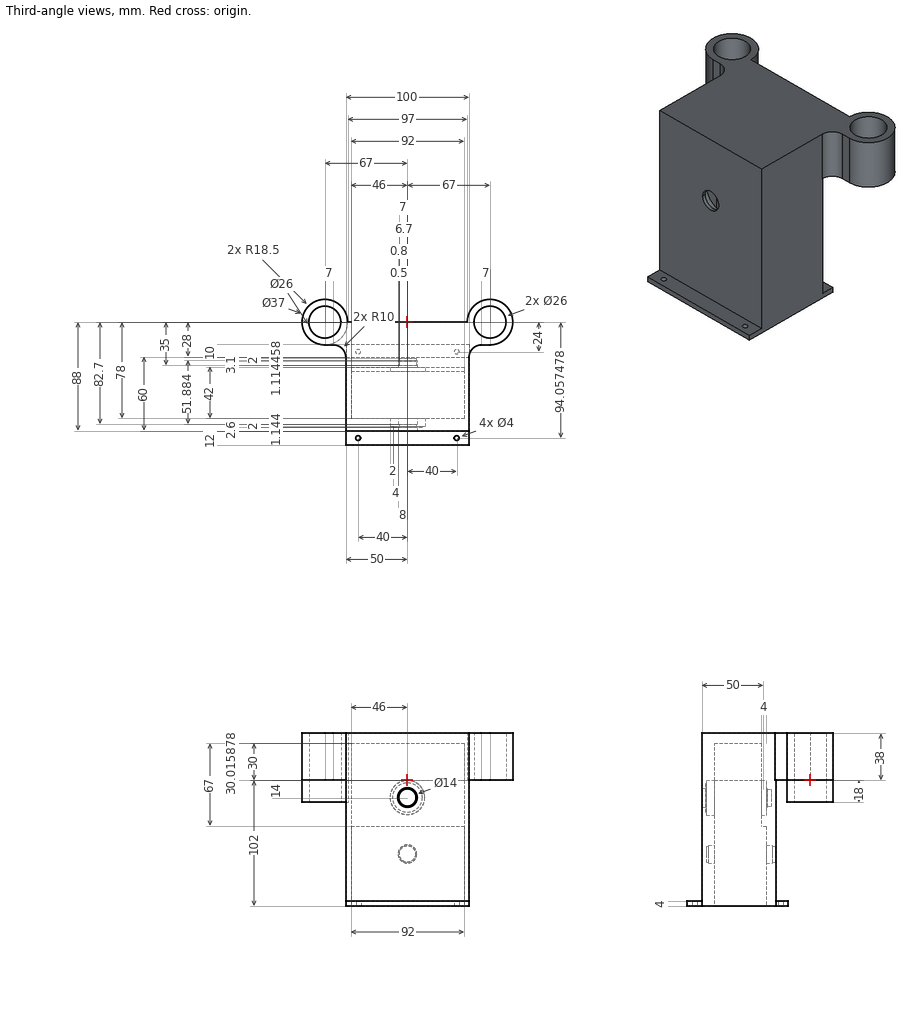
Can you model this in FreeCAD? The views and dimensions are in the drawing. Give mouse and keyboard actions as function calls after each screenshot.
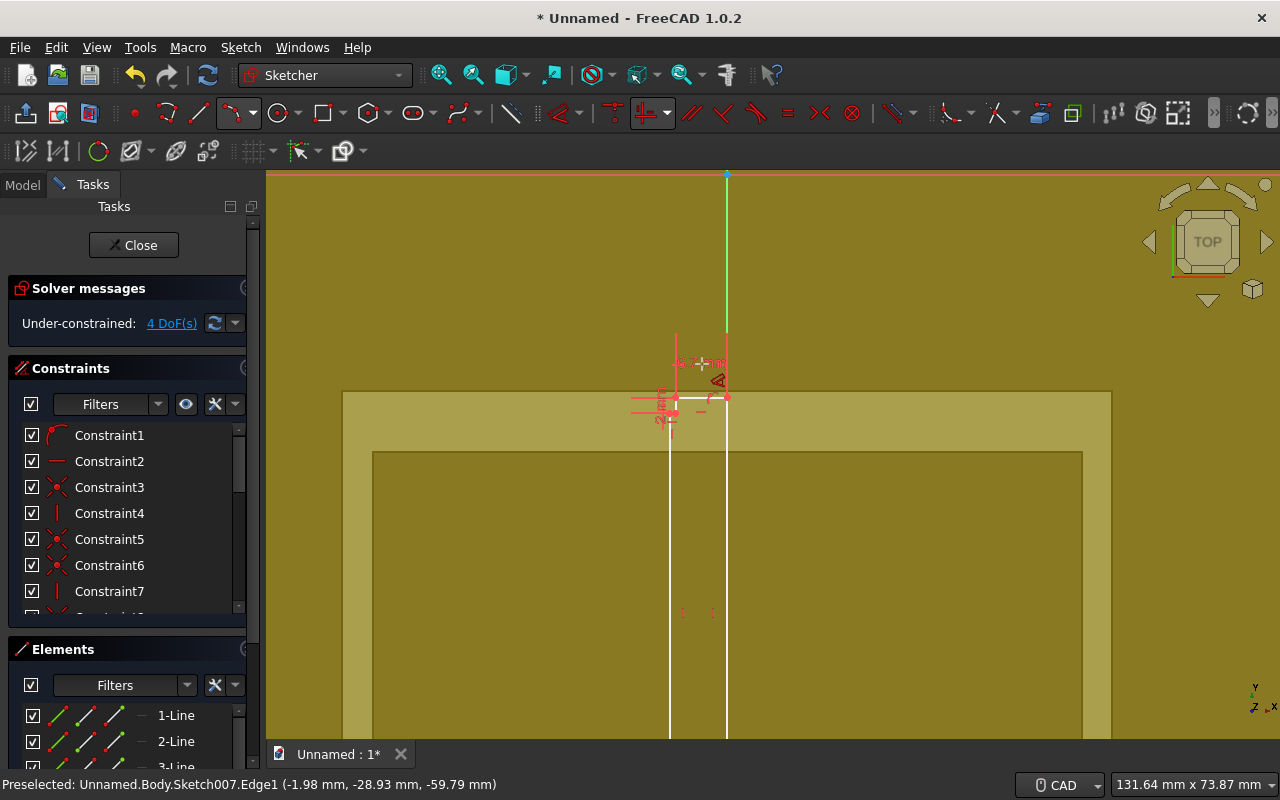
scroll(673, 413, up, 10)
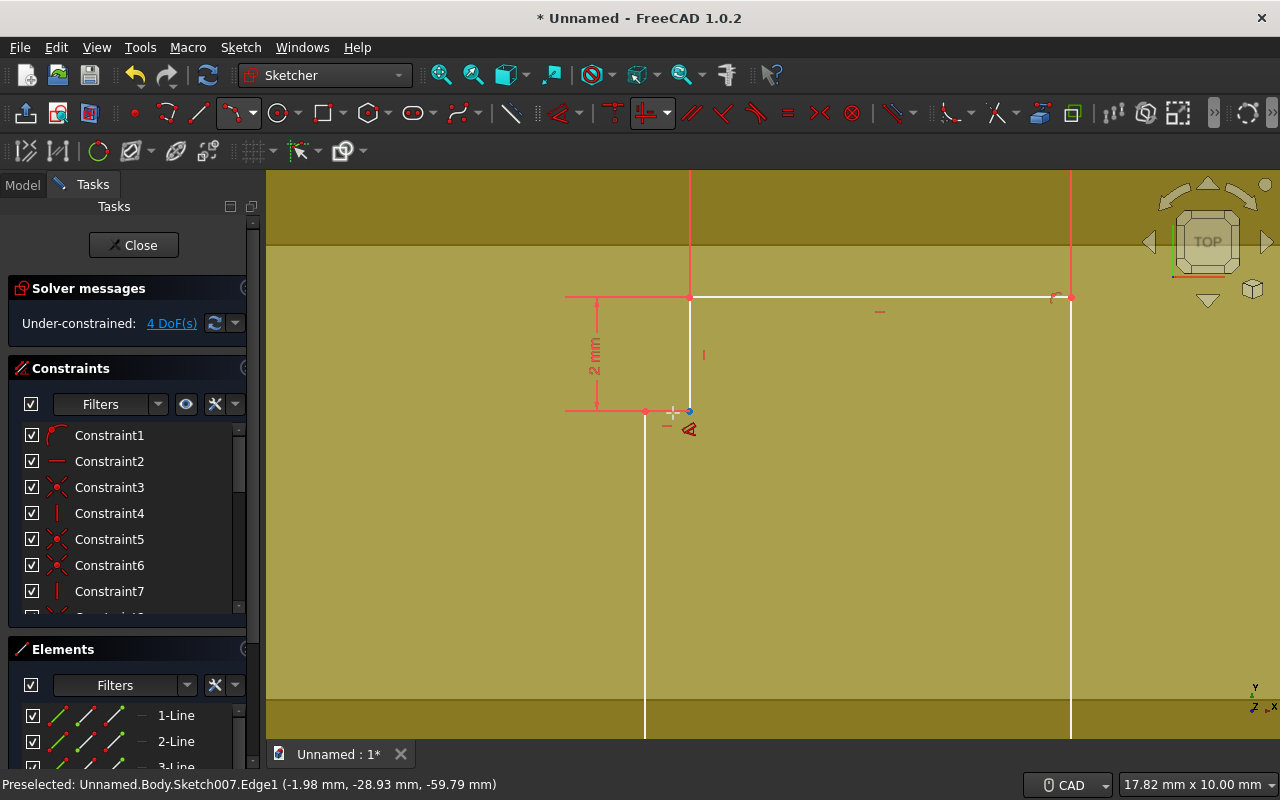
click(668, 411)
click(668, 377)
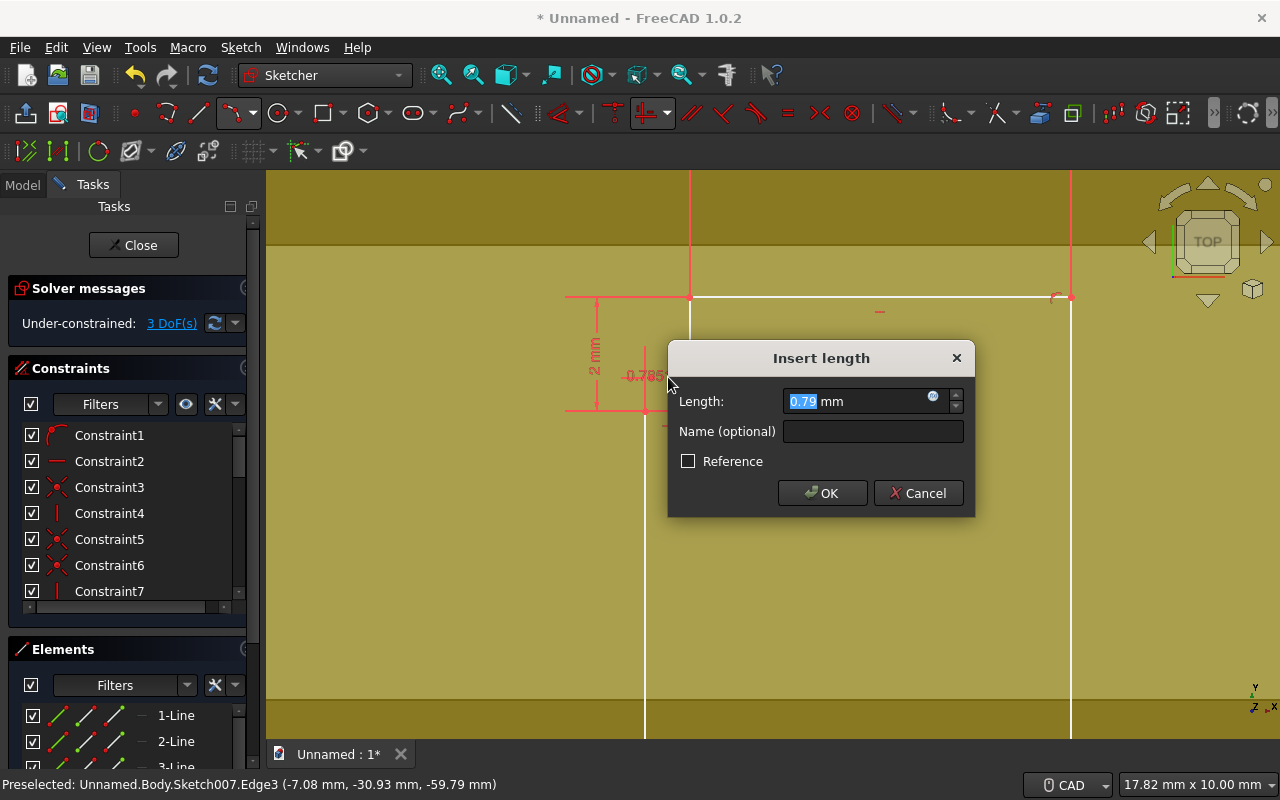
text(0.8)
key(Return)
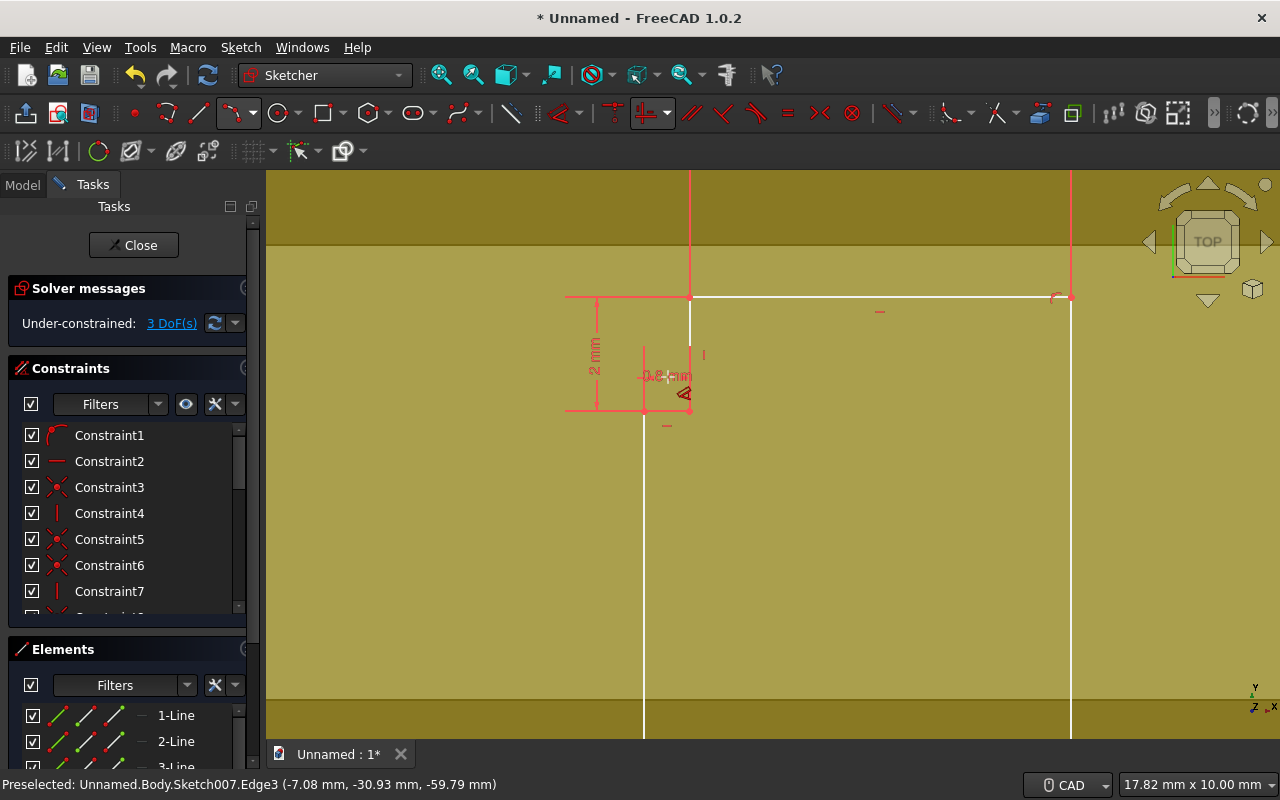
scroll(692, 406, down, 13)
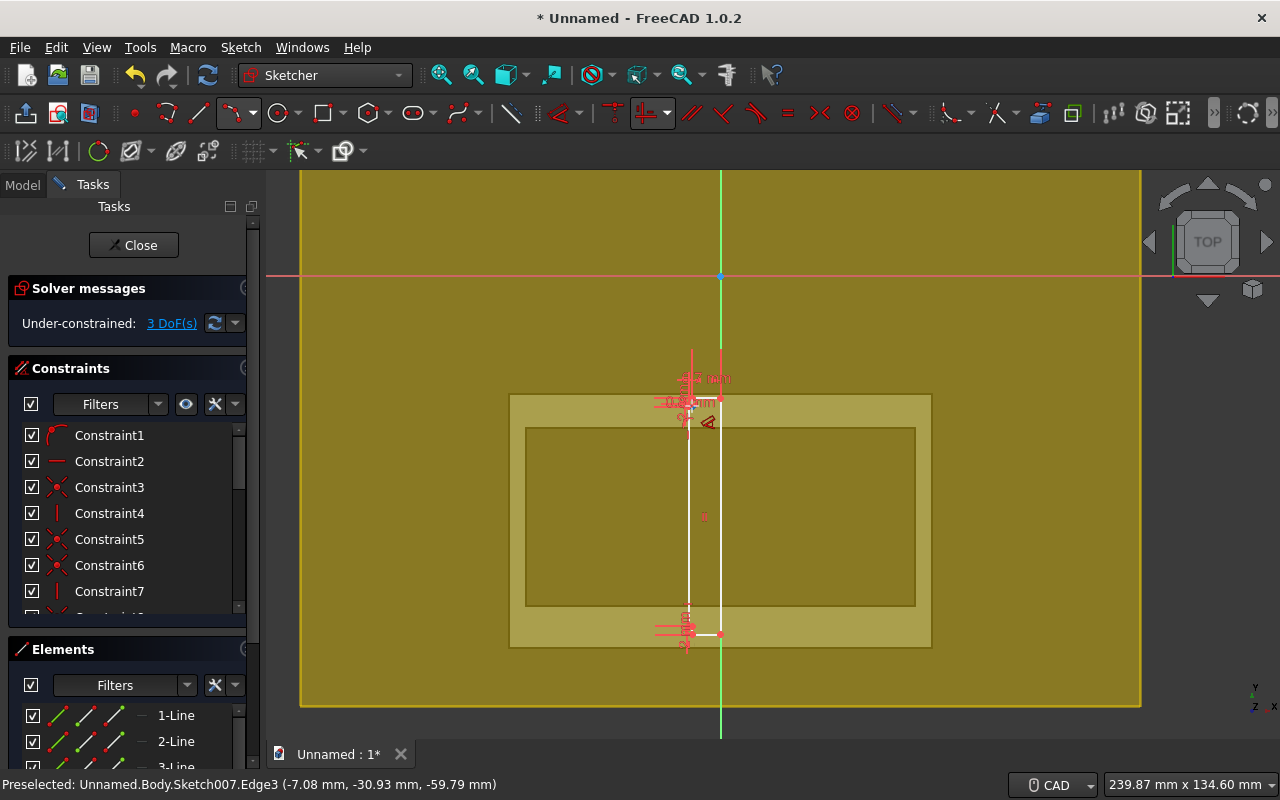
scroll(690, 626, up, 13)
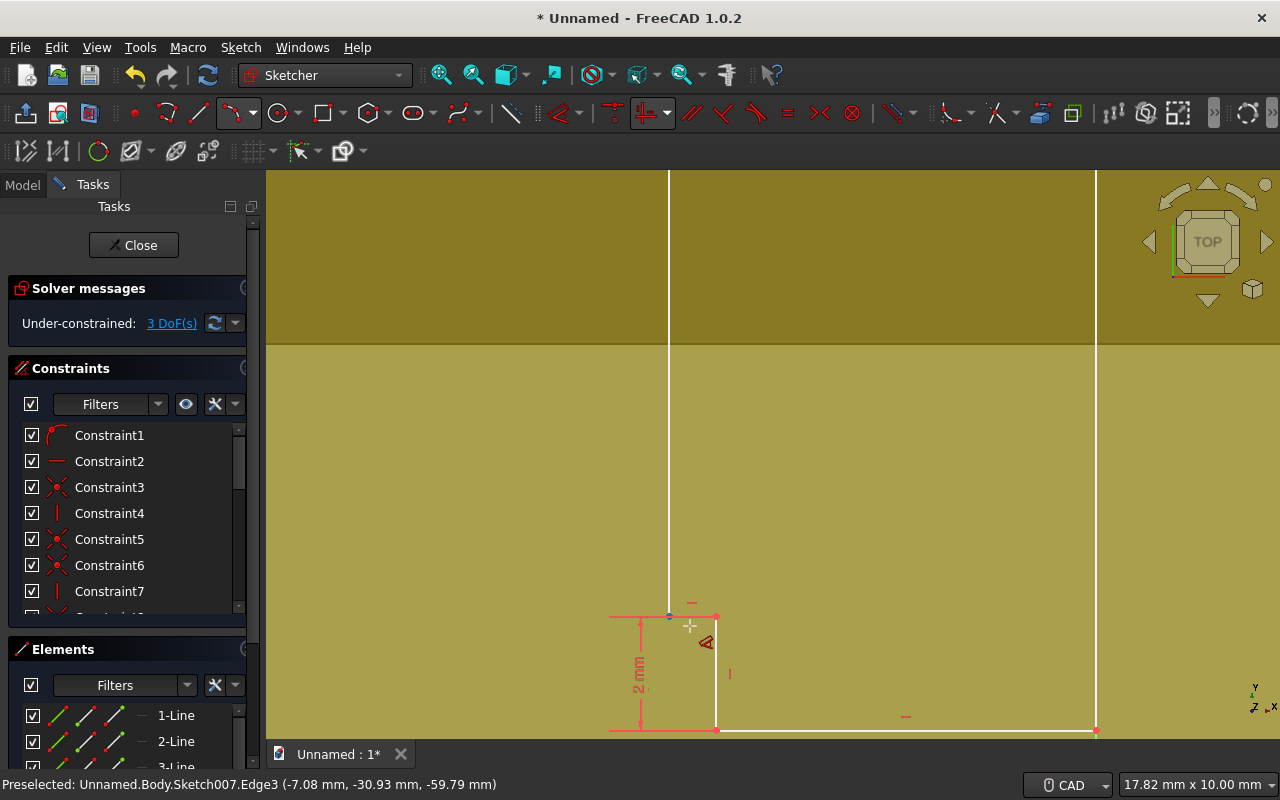
click(683, 617)
click(693, 651)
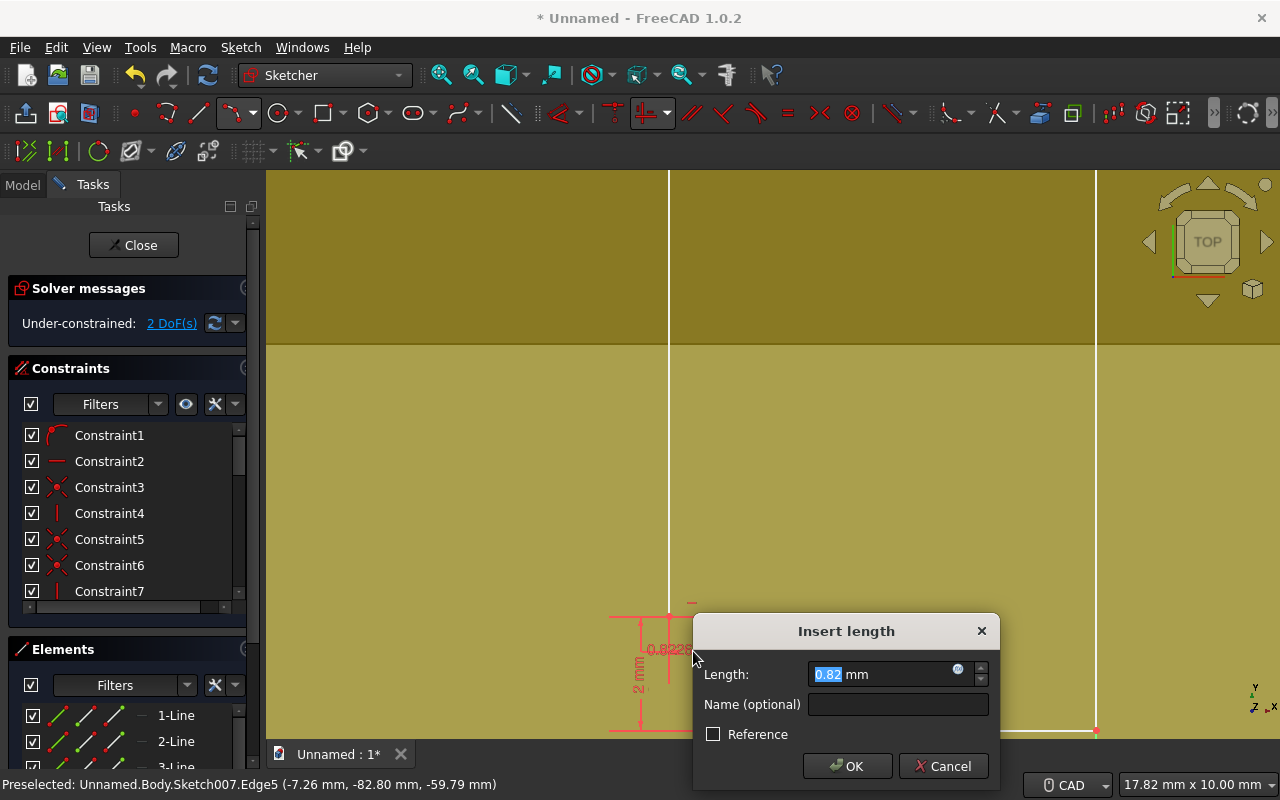
text(0.8)
key(Return)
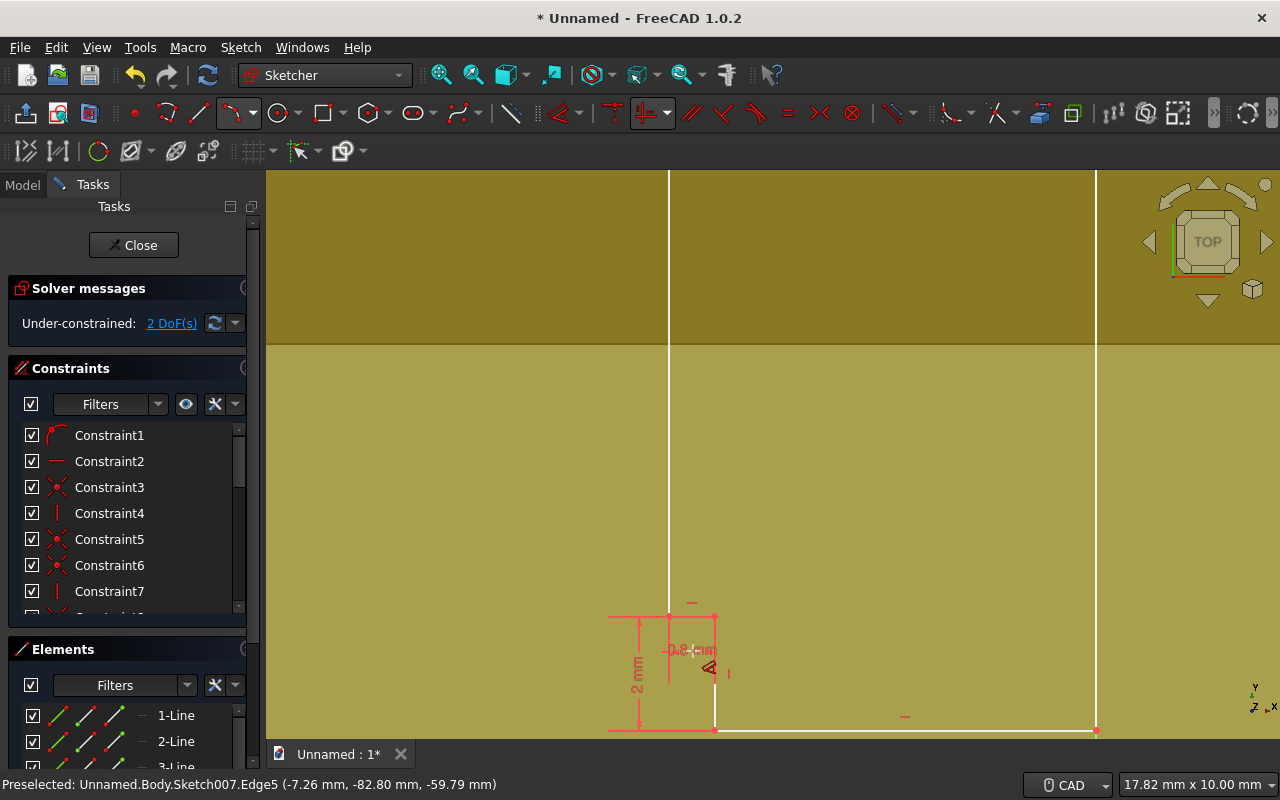
scroll(690, 626, down, 13)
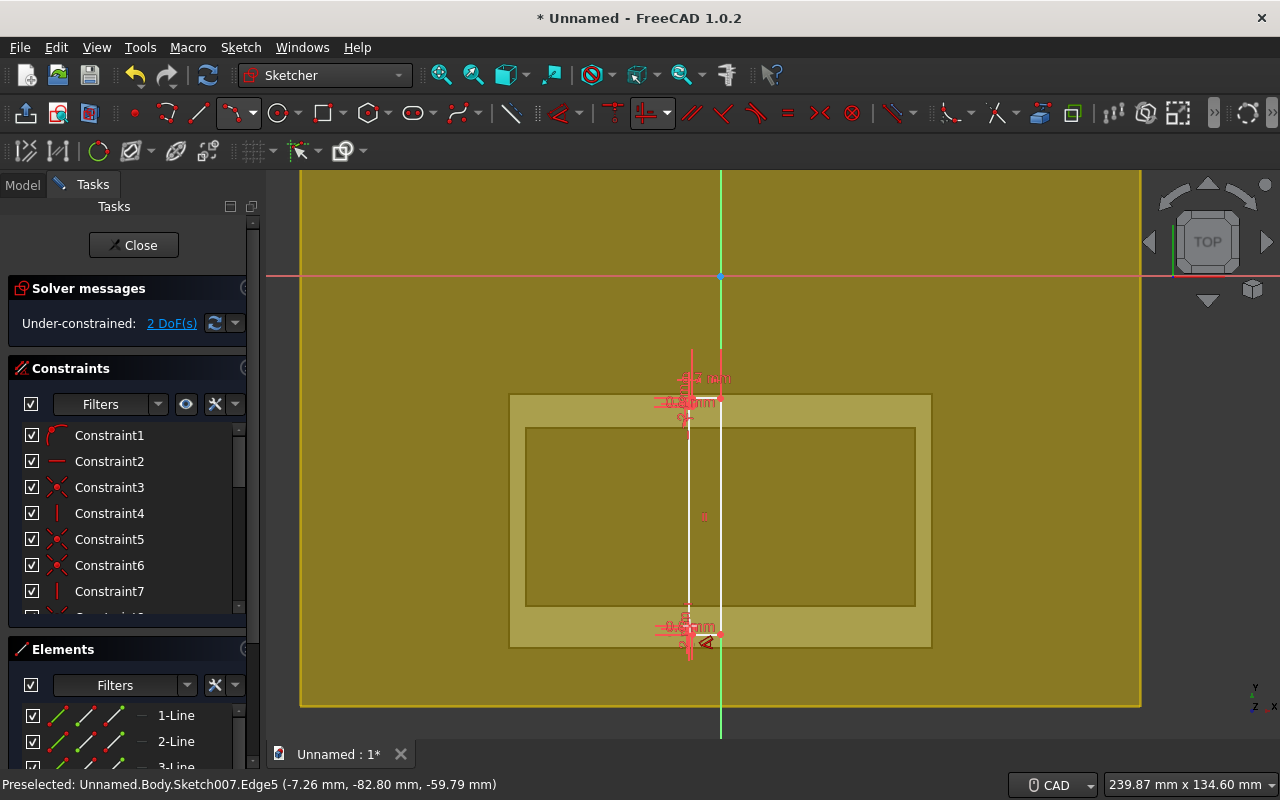
scroll(689, 626, up, 7)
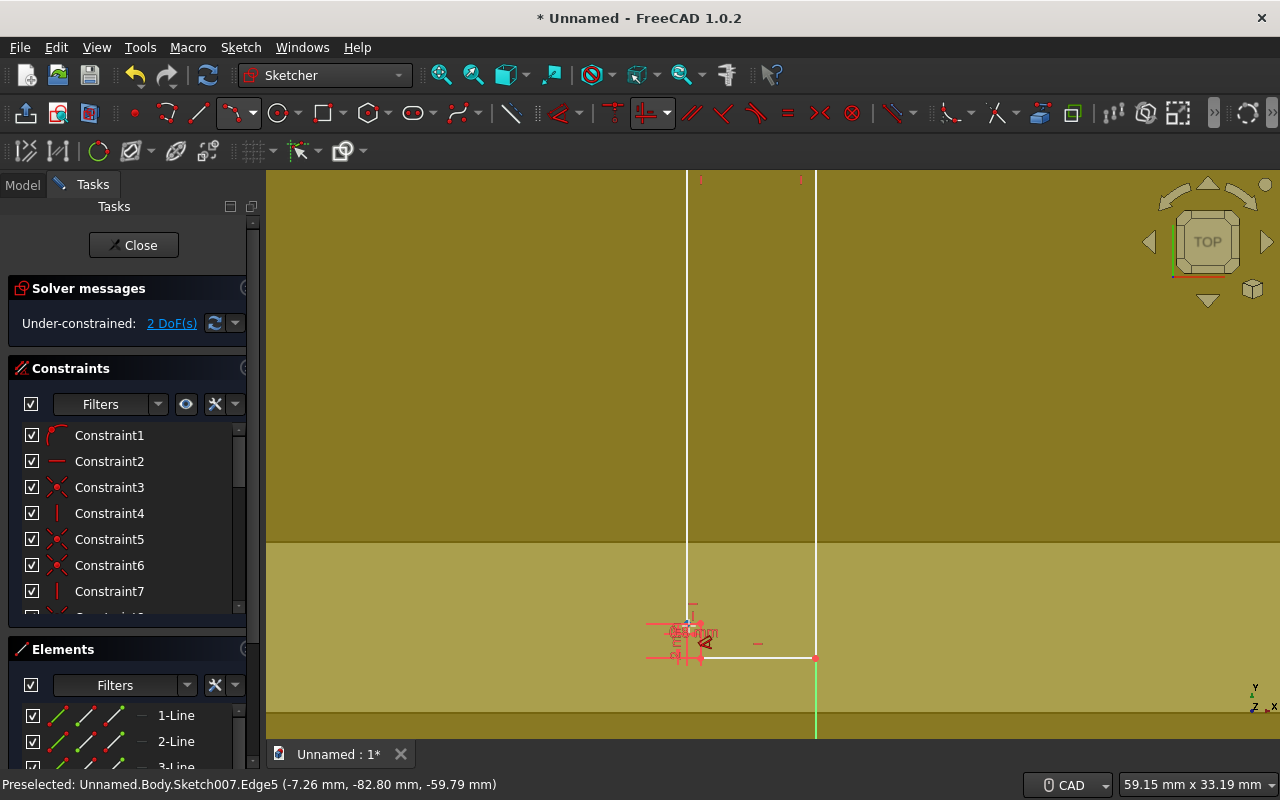
click(687, 624)
click(850, 411)